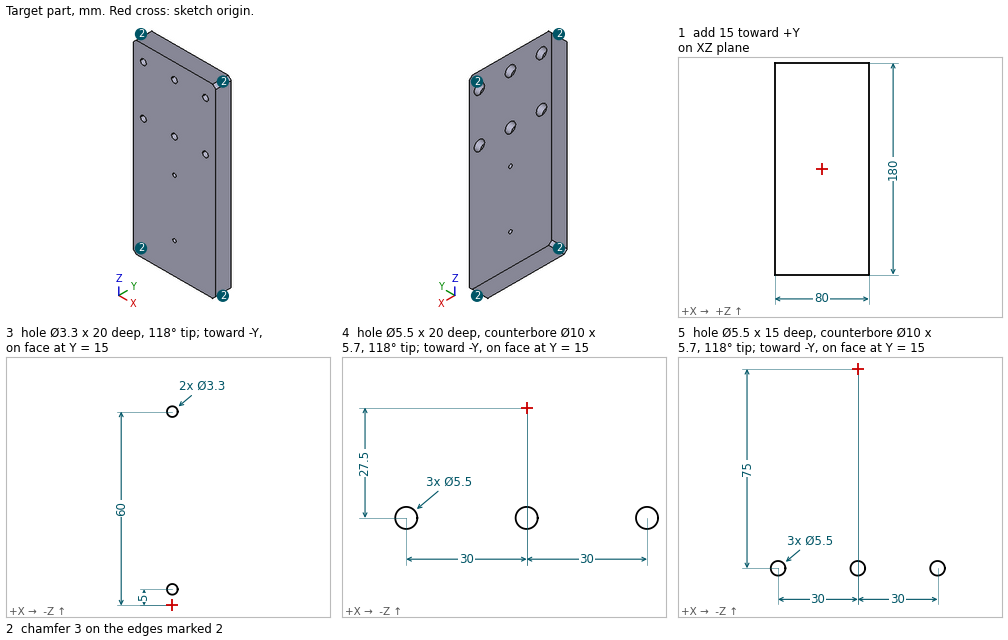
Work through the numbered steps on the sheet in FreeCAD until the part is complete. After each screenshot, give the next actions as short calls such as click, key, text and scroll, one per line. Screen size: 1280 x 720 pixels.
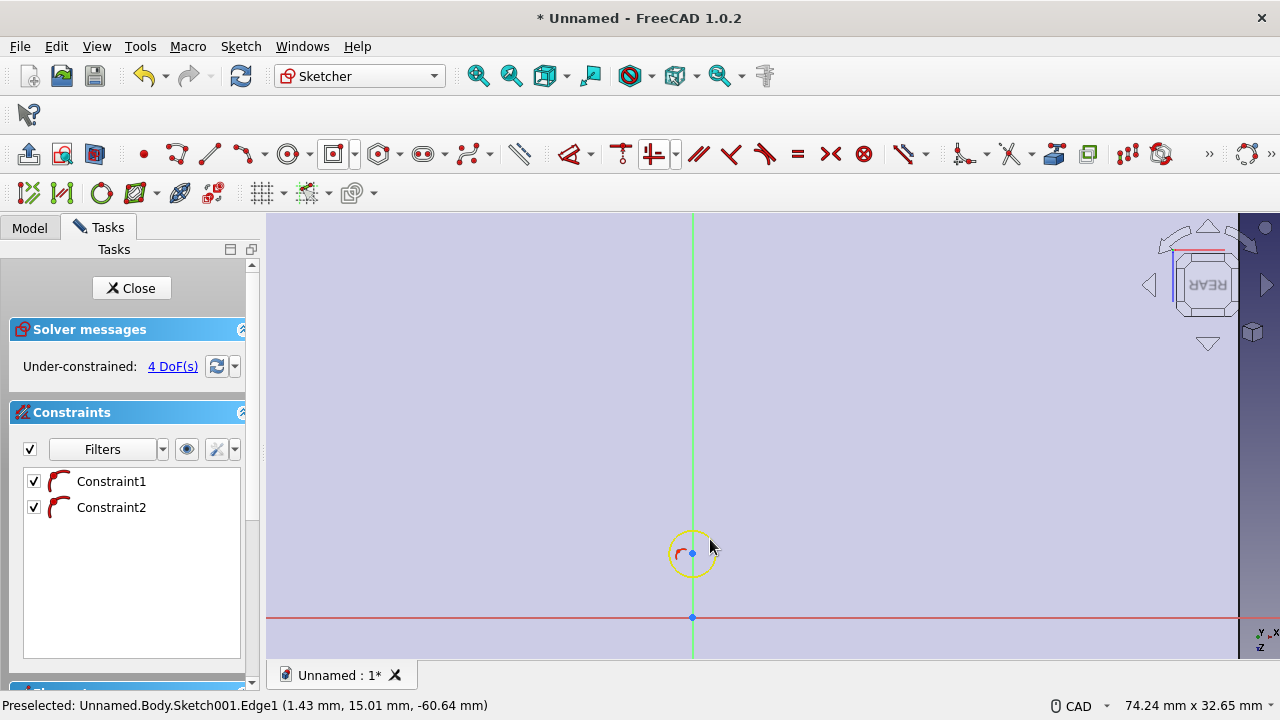
click(709, 537)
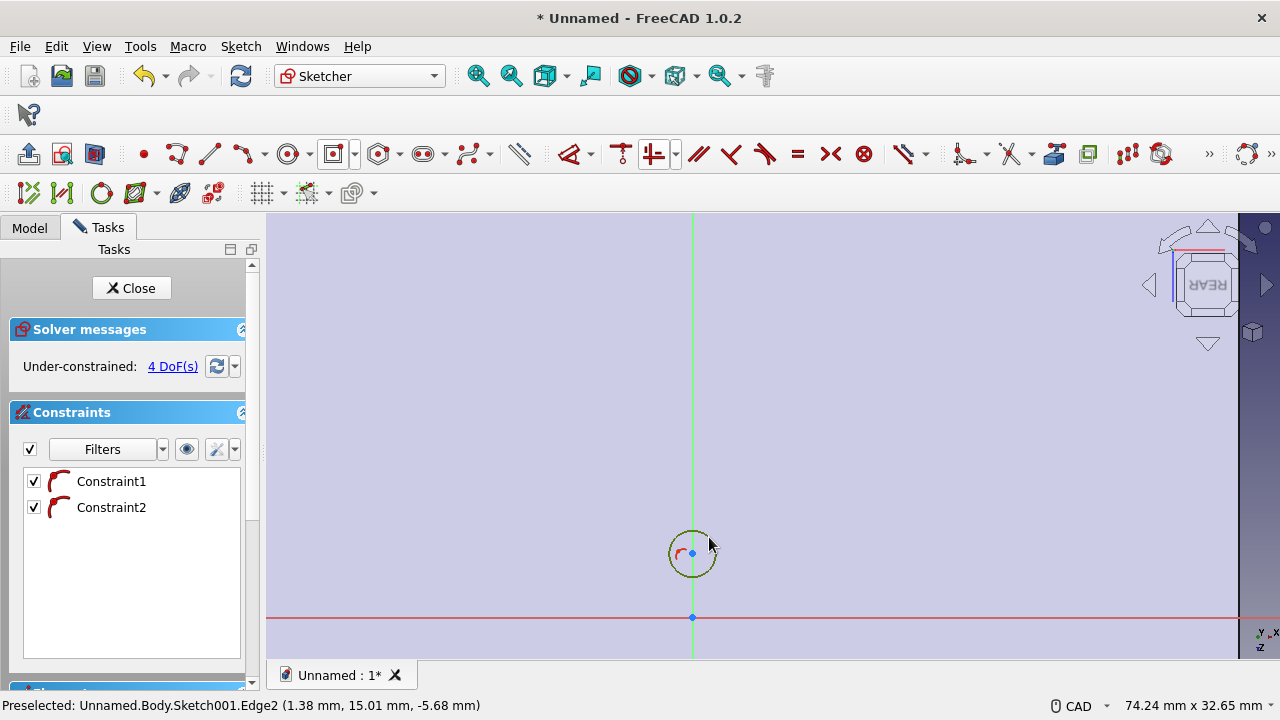
click(798, 154)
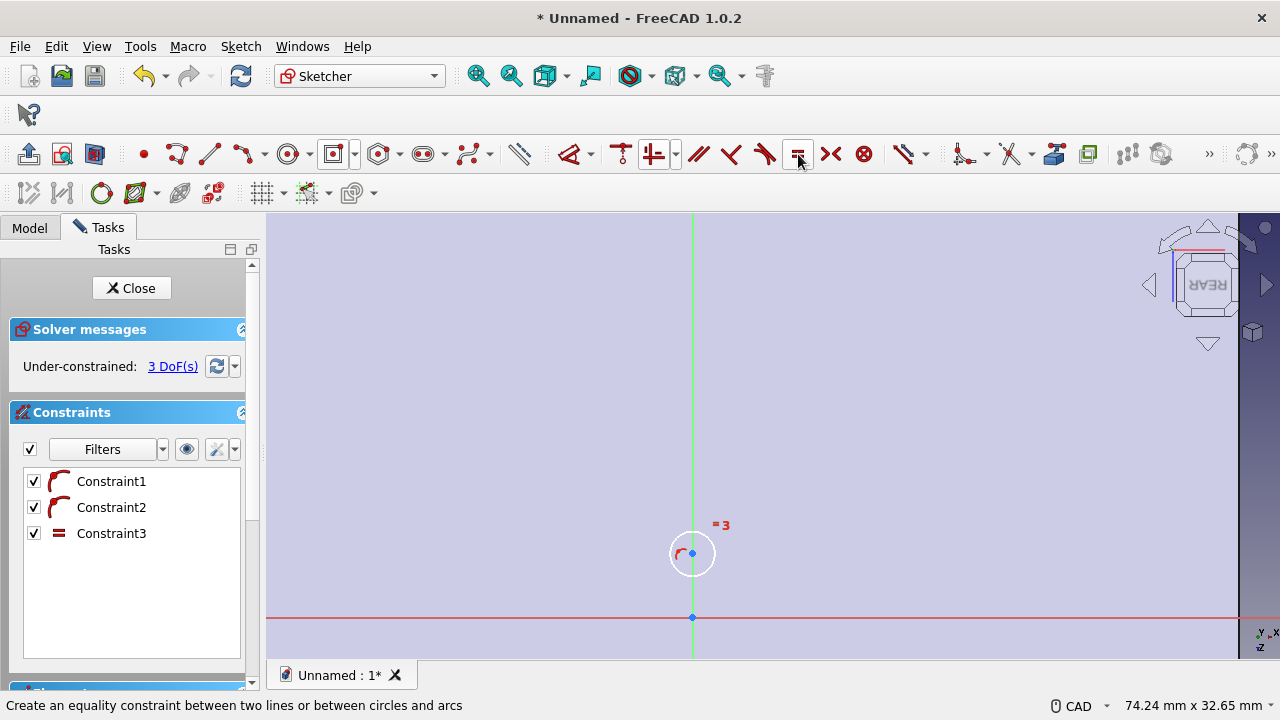
click(568, 154)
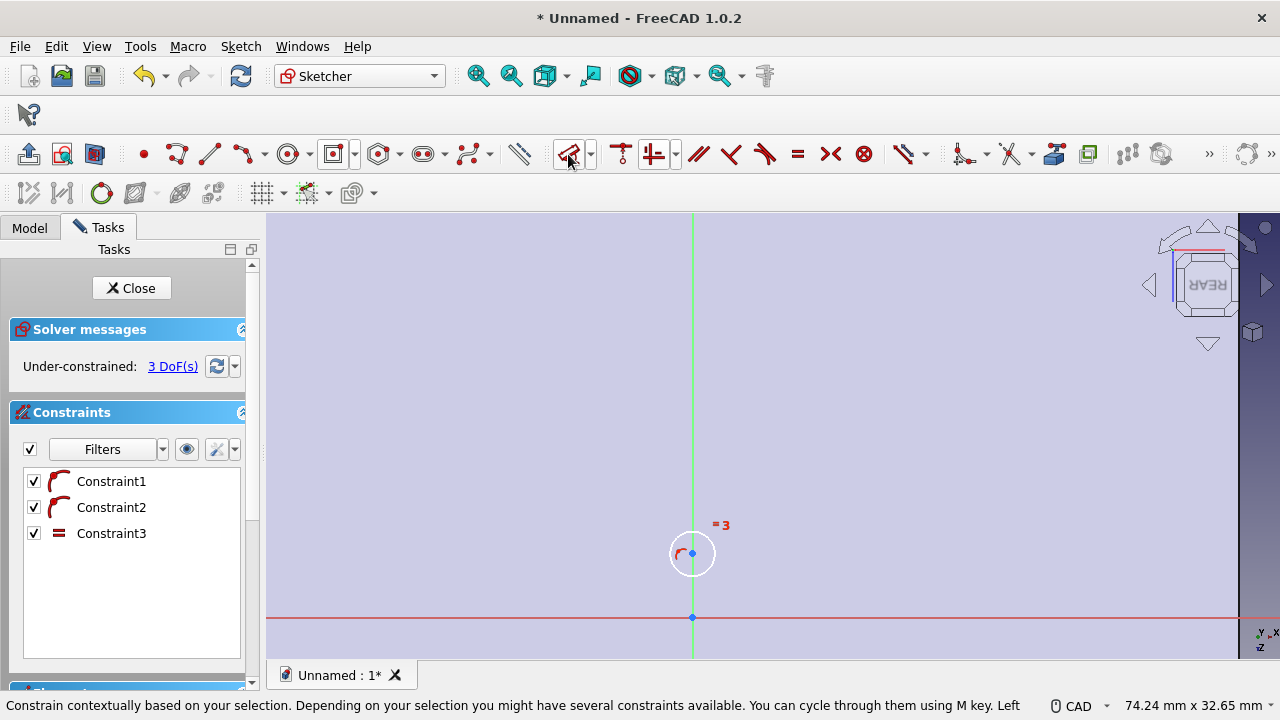
scroll(710, 539, down, 6)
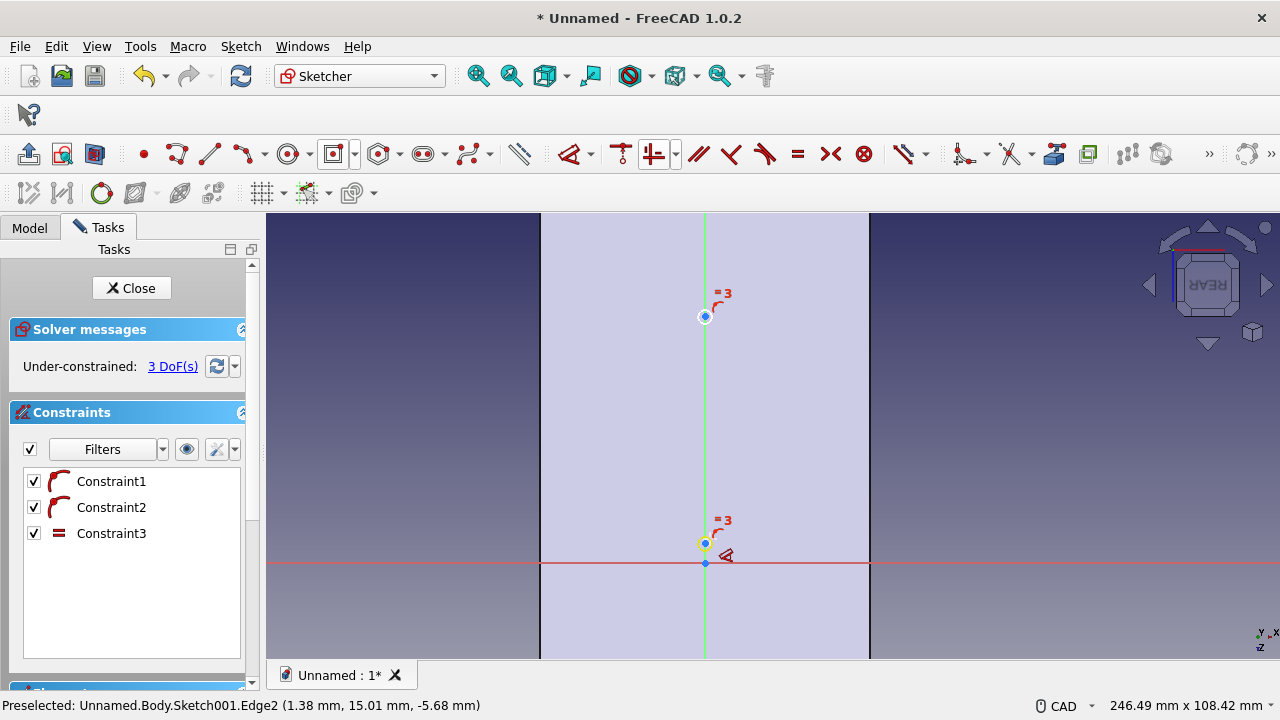
scroll(710, 312, up, 6)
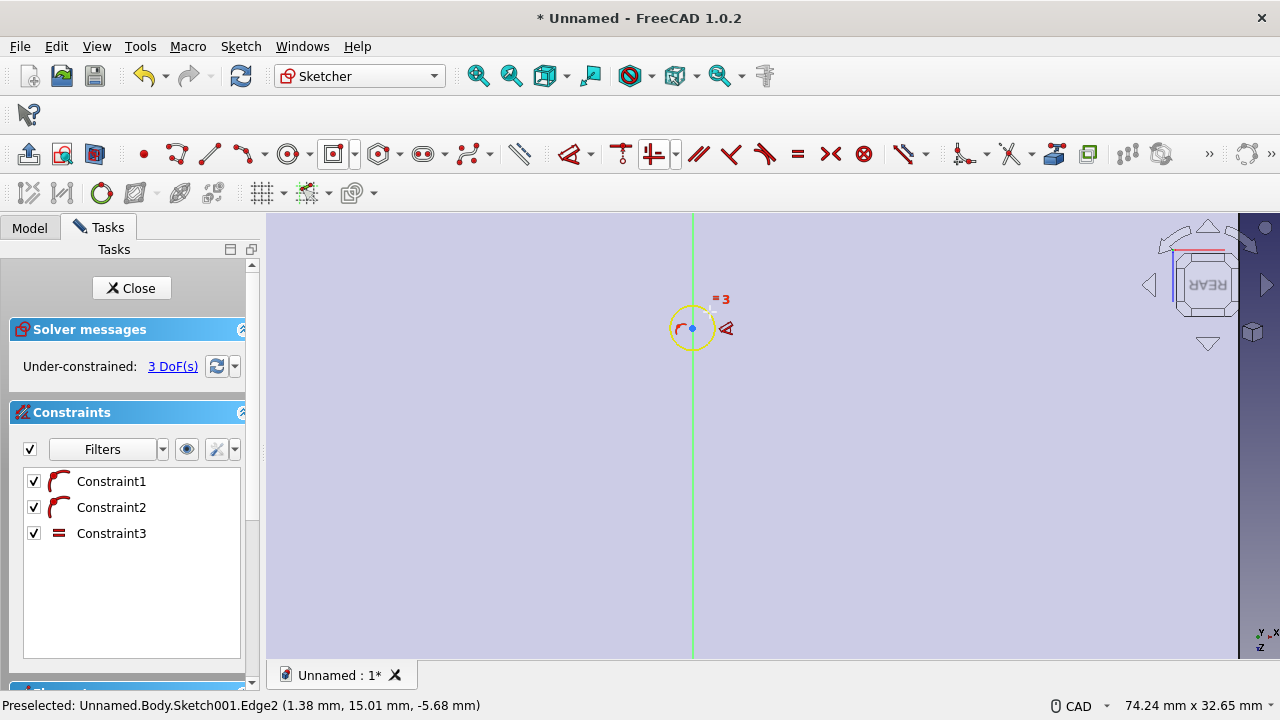
click(708, 312)
click(730, 289)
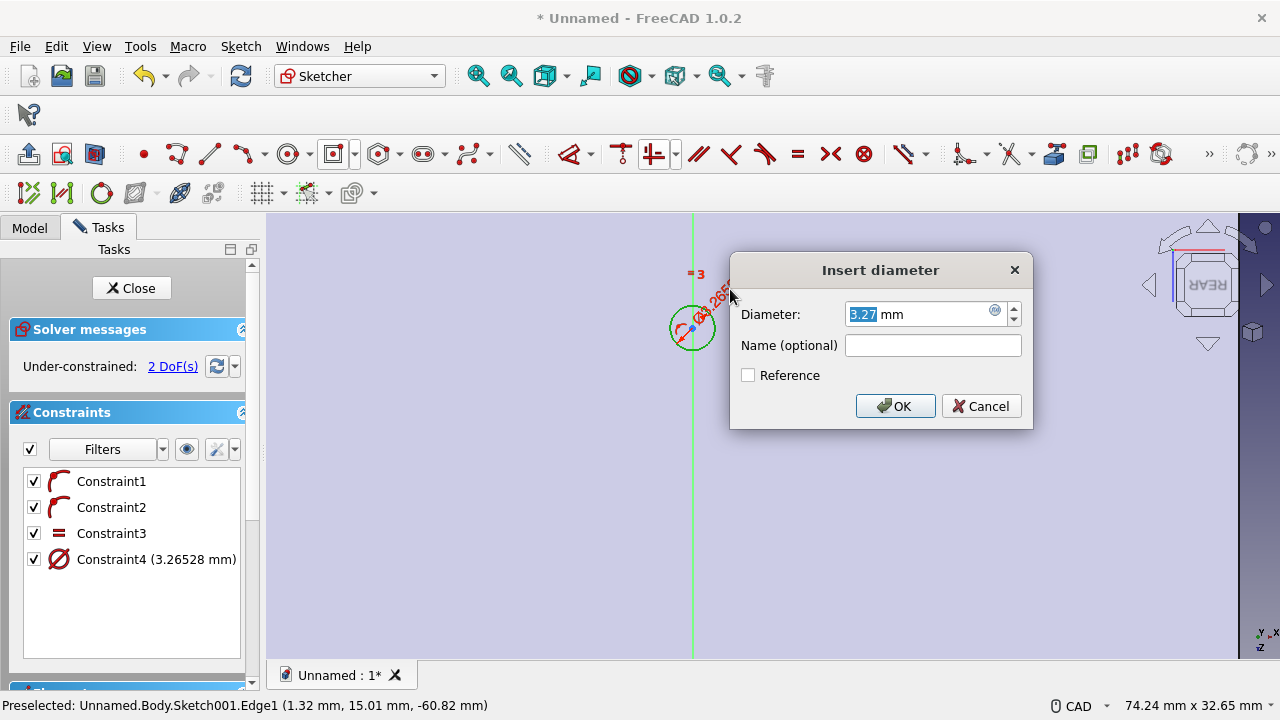
text(3.3)
key(Return)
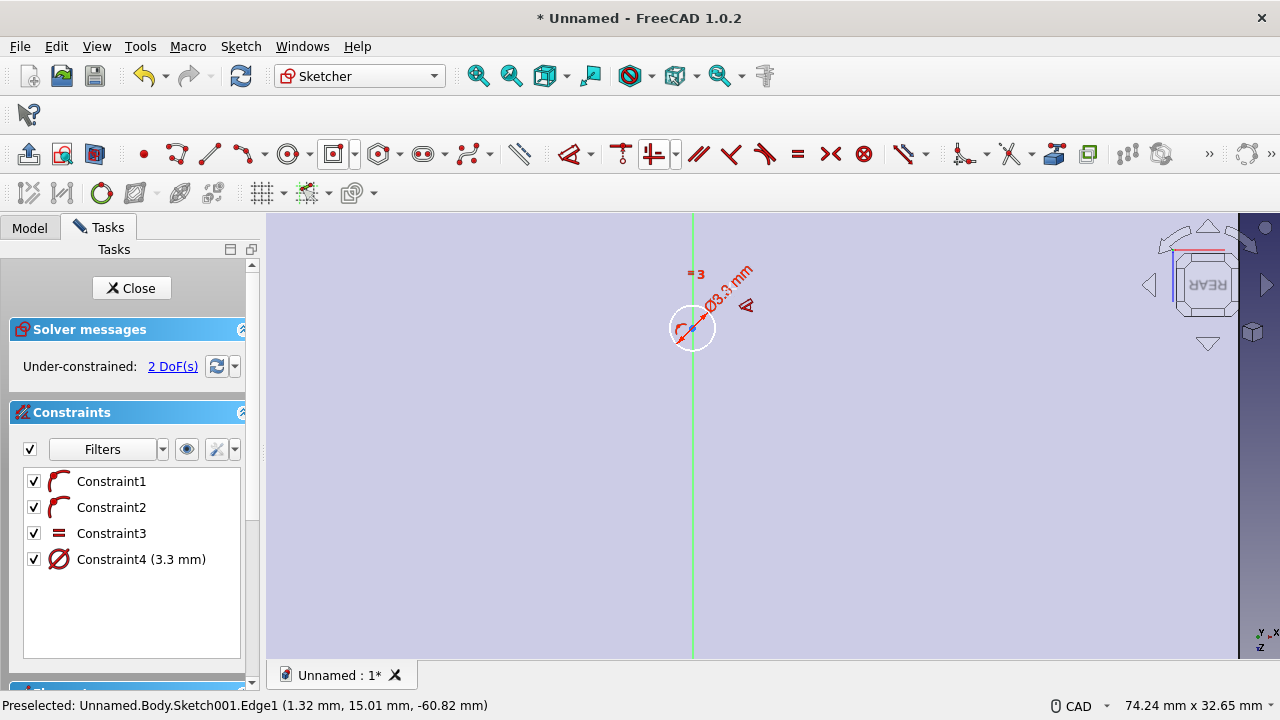
scroll(710, 312, down, 6)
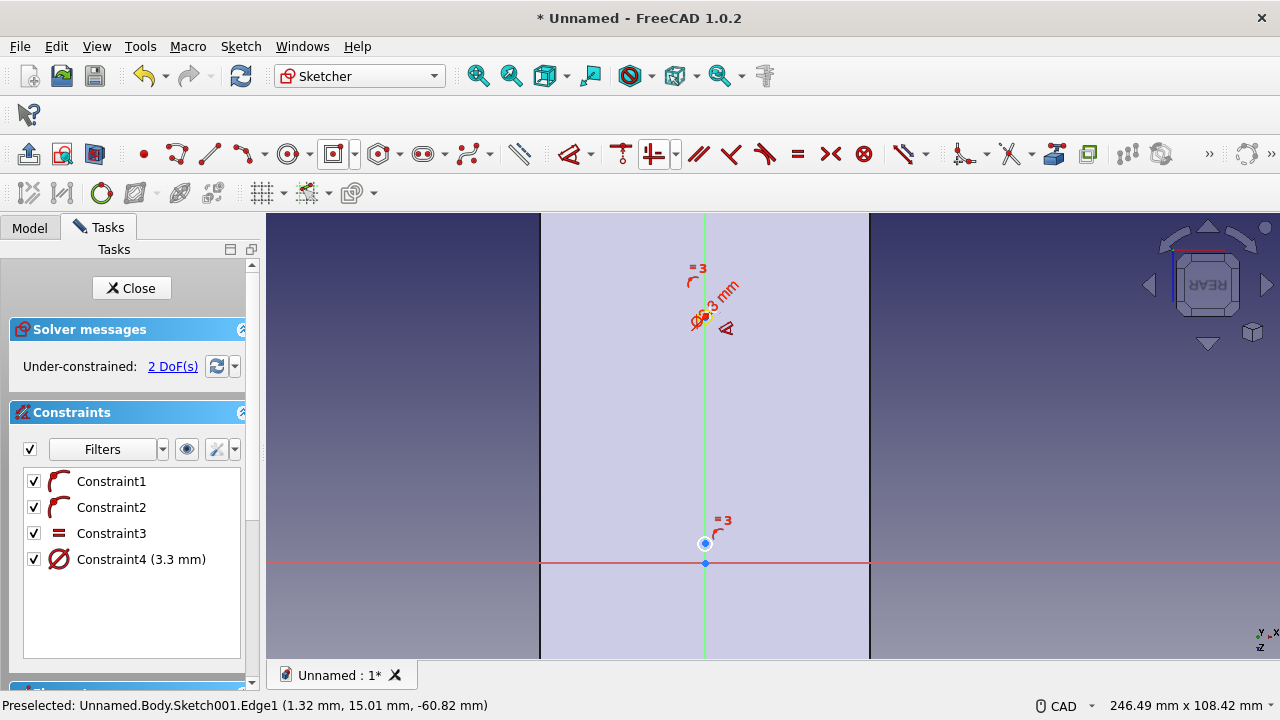
scroll(705, 544, up, 4)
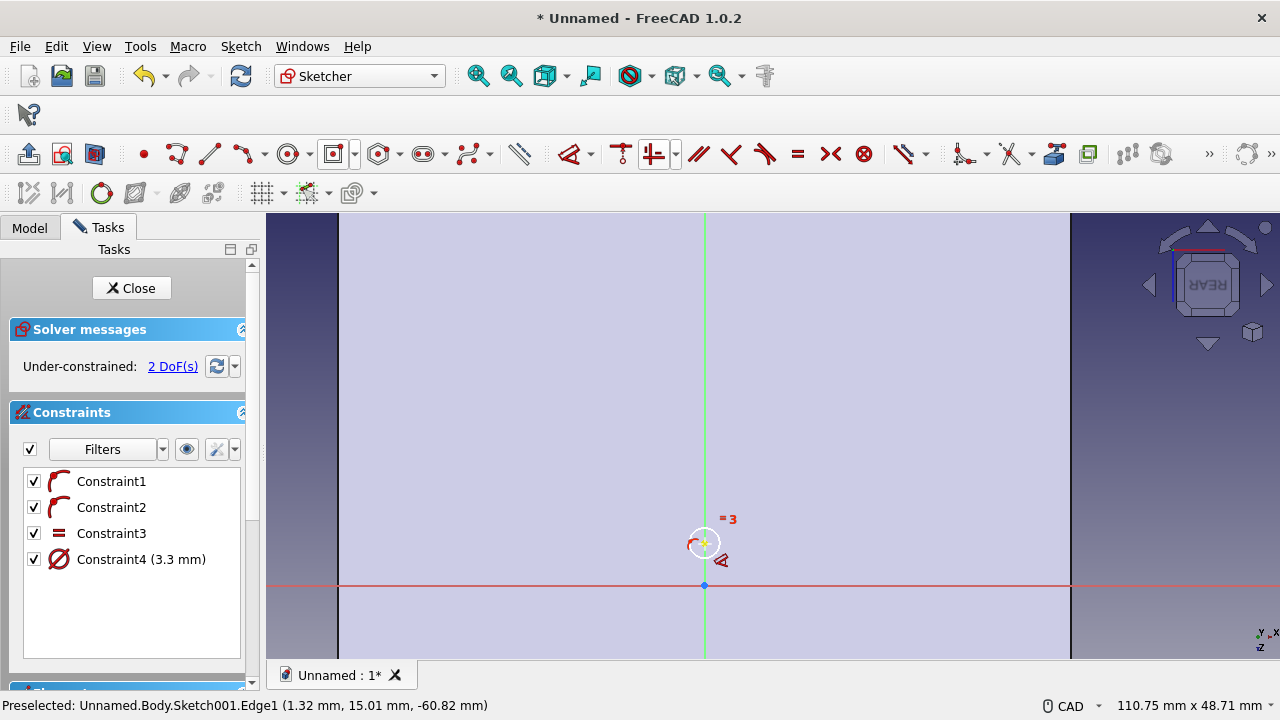
click(705, 543)
click(739, 564)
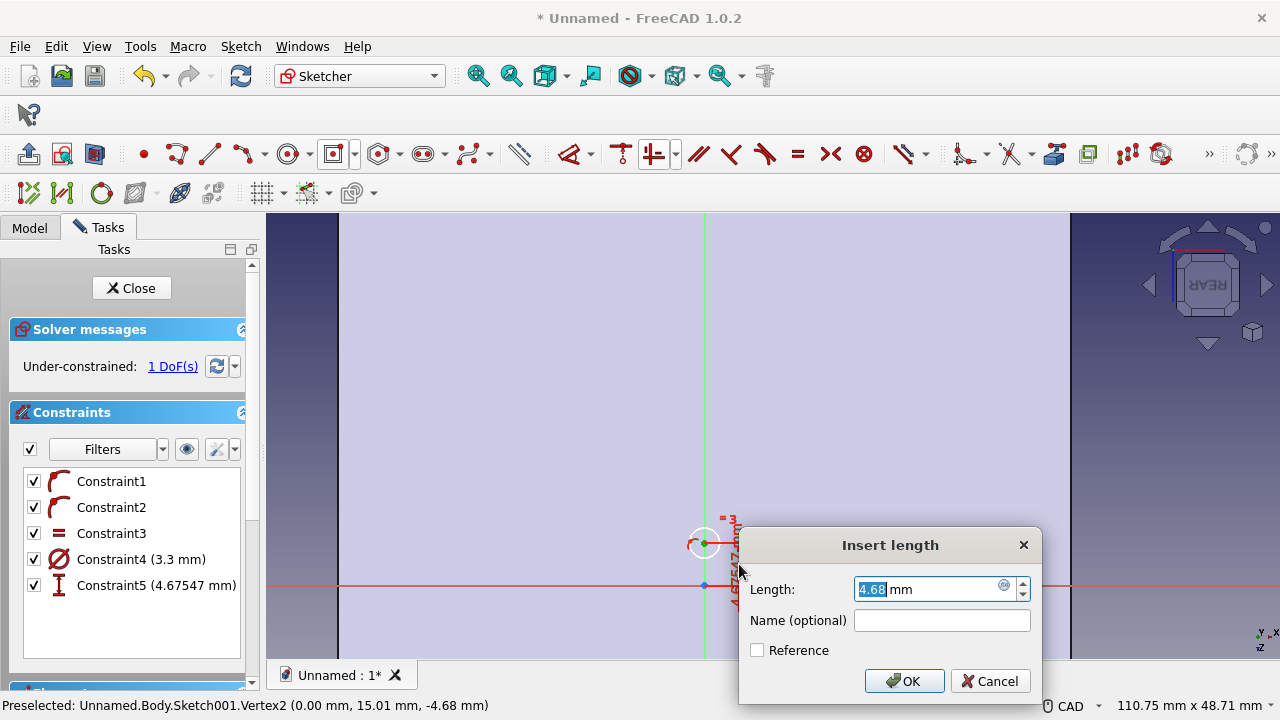
text(5)
key(Return)